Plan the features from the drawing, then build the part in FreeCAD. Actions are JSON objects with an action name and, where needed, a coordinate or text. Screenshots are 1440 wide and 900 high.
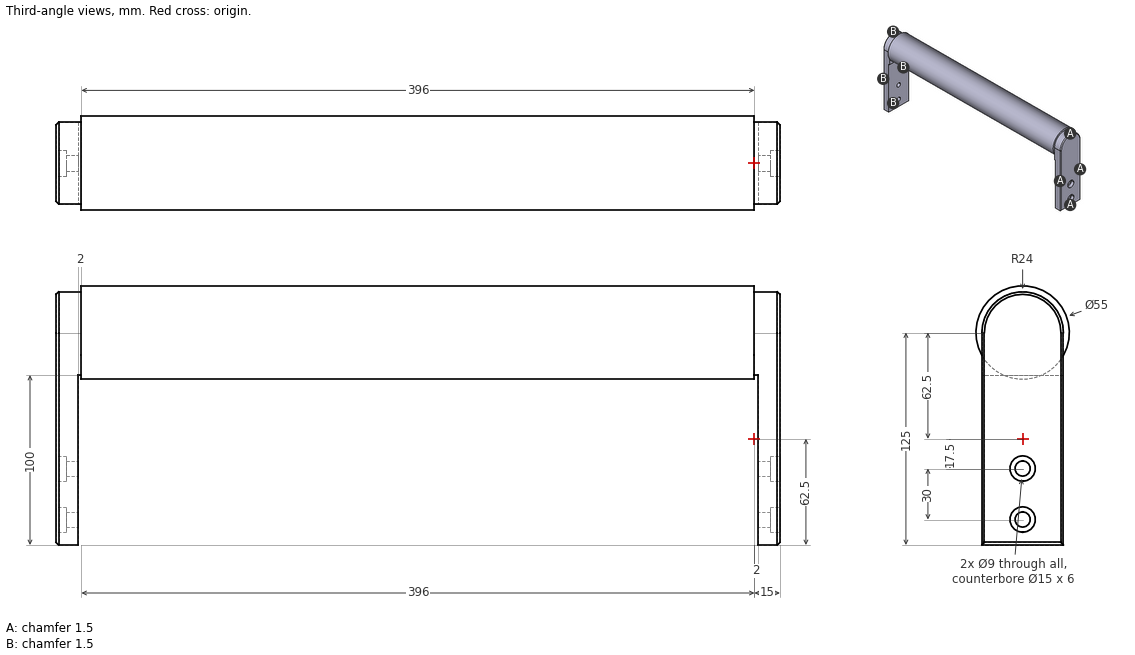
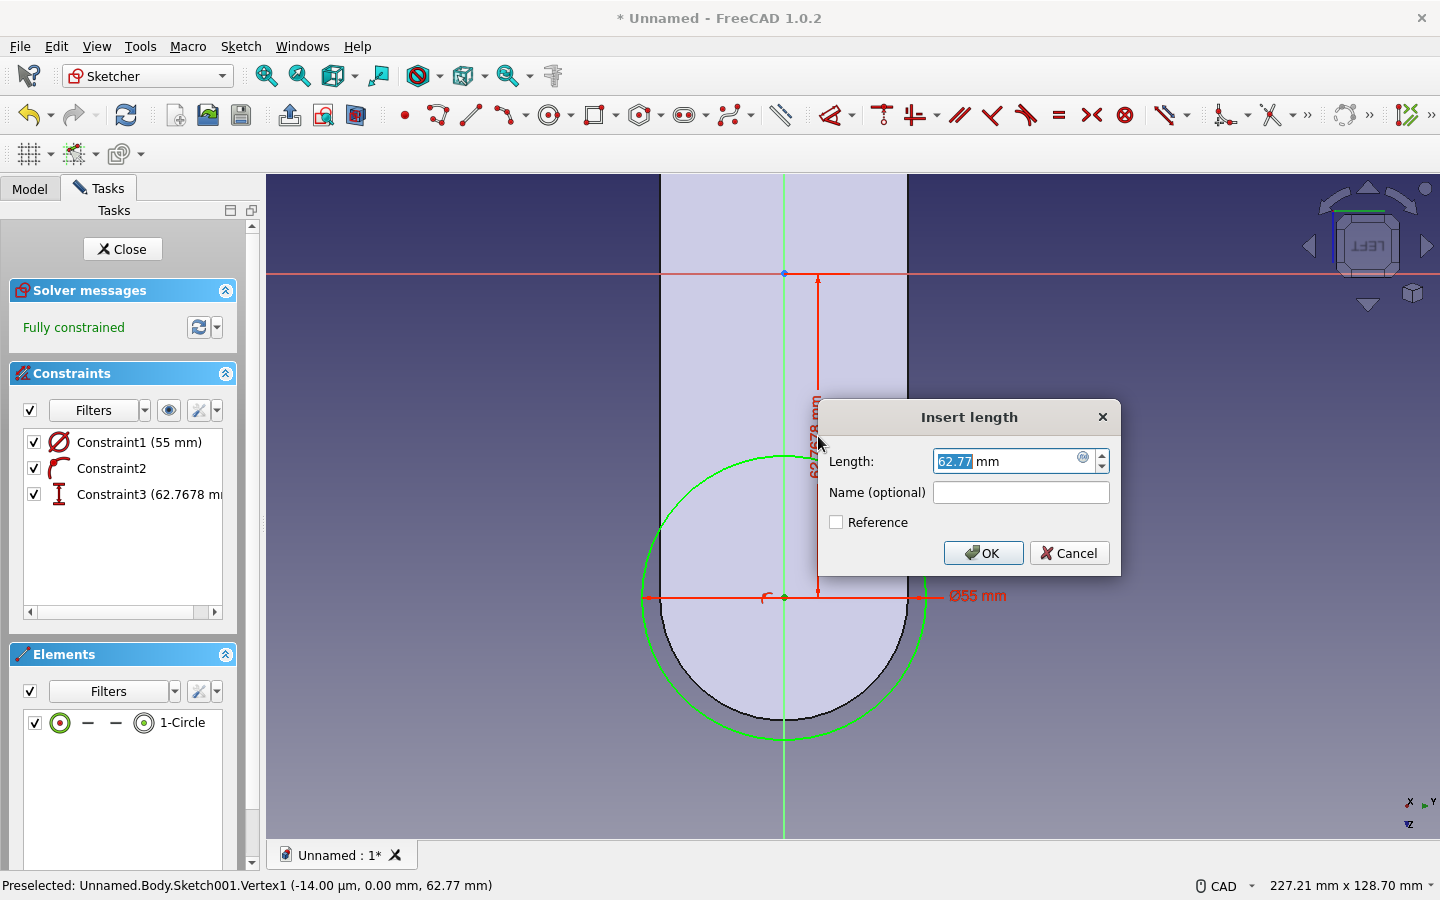
{"action": "type", "text": "62.5"}
{"action": "key", "text": "Return"}
{"action": "key", "text": "Escape"}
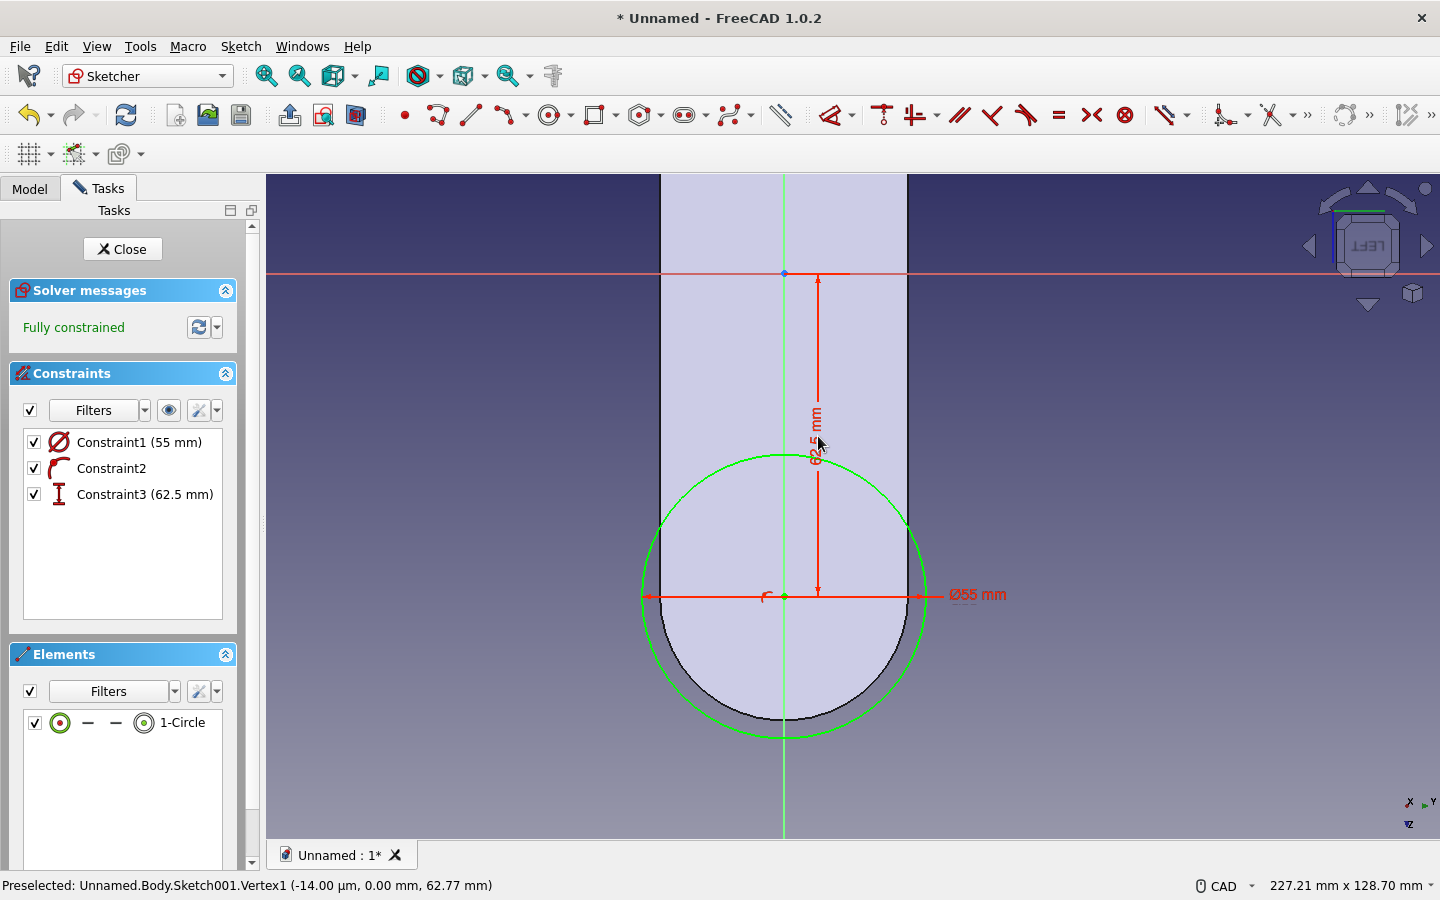
{"action": "left_click", "coordinate": [123, 249]}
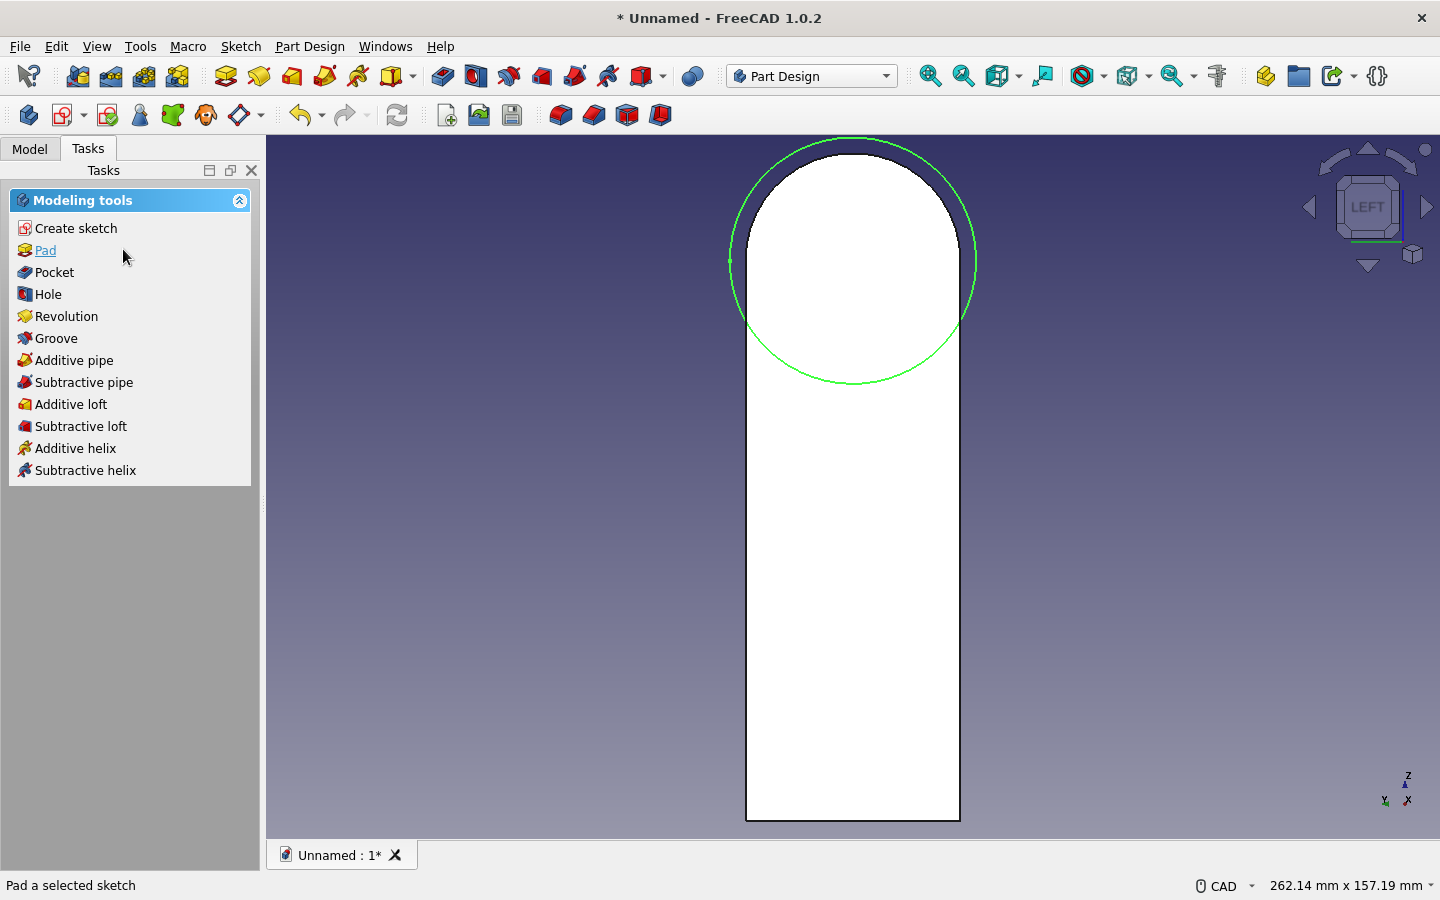
{"action": "left_click", "coordinate": [226, 76]}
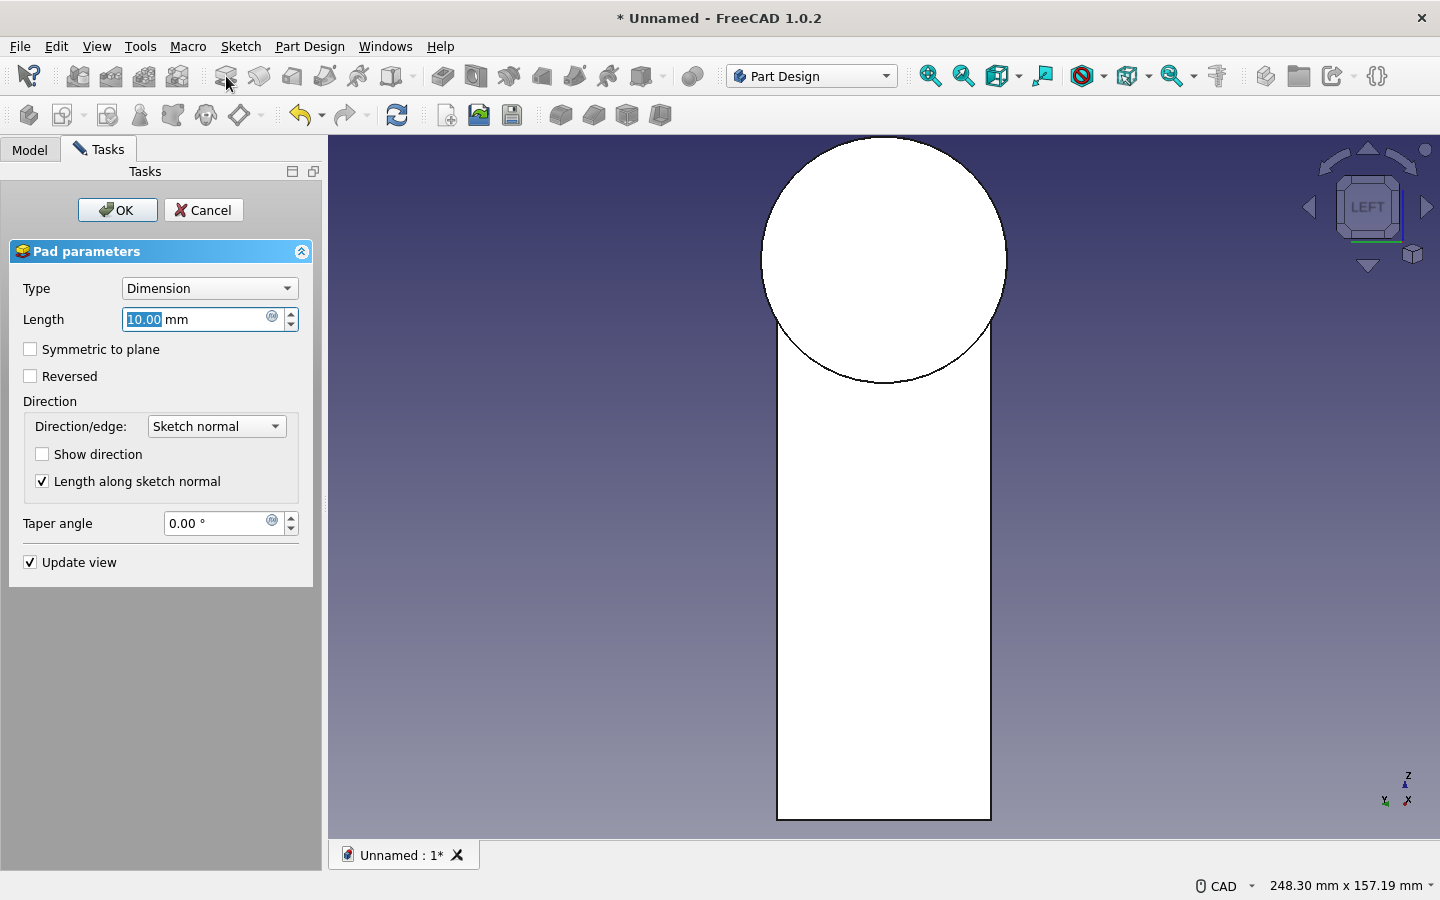
{"action": "type", "text": "396"}
{"action": "key", "text": "Tab"}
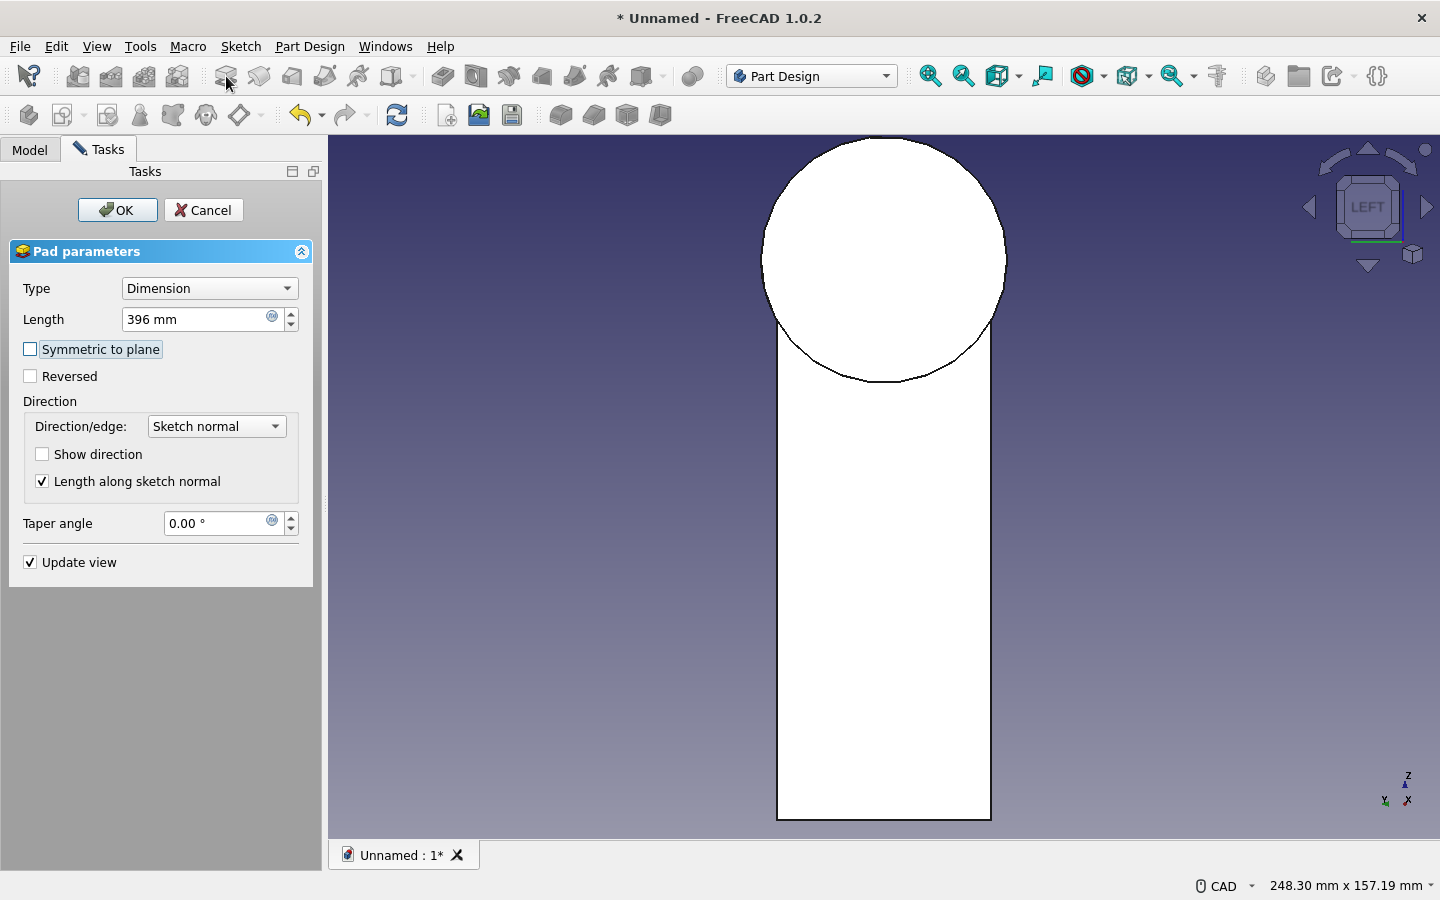
{"action": "left_click", "coordinate": [118, 210]}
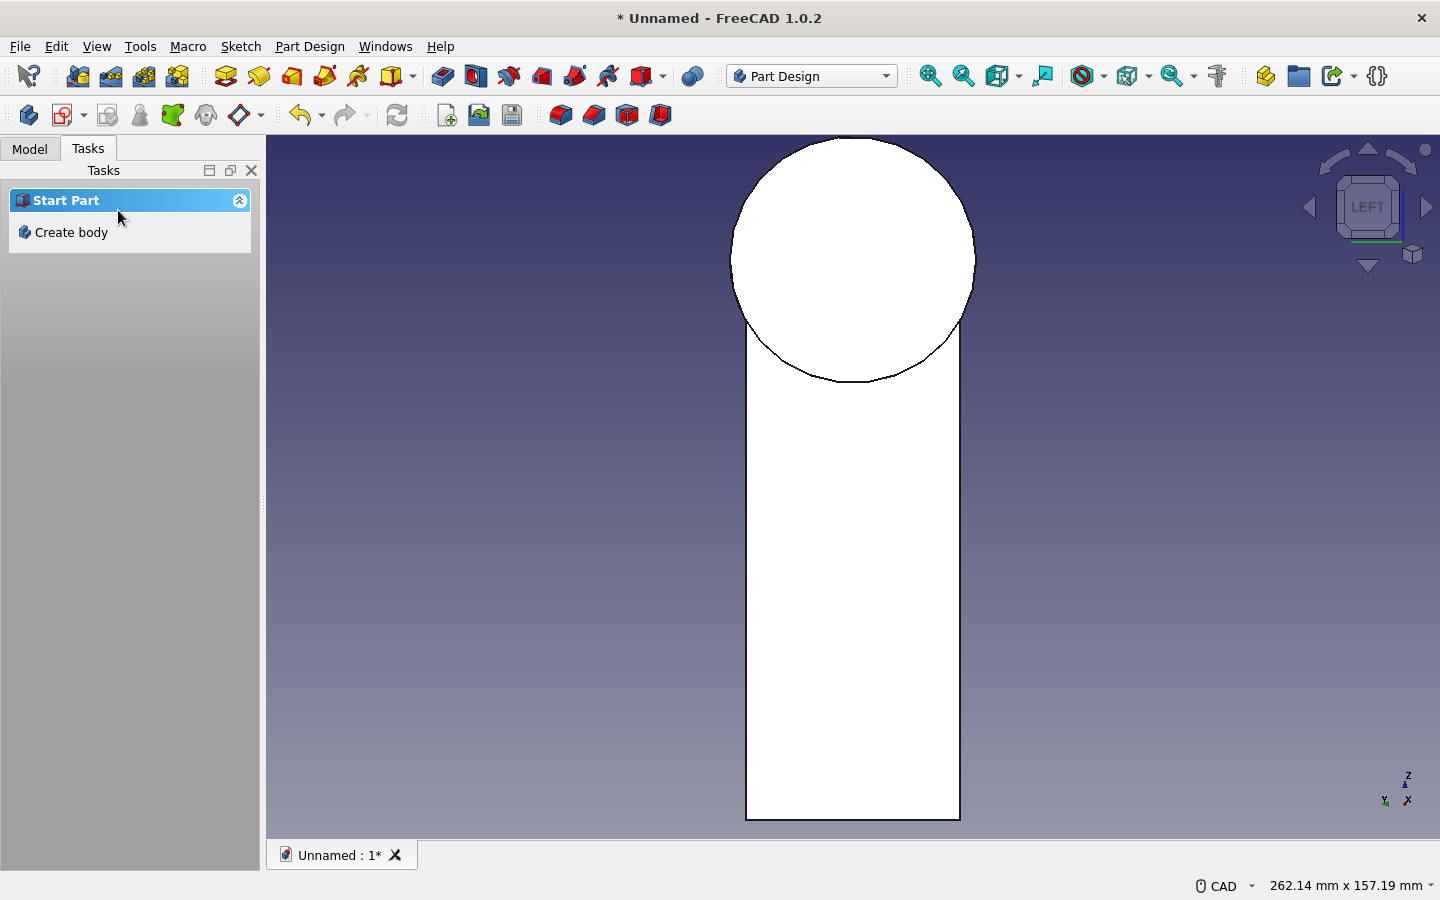
{"action": "key", "text": "0"}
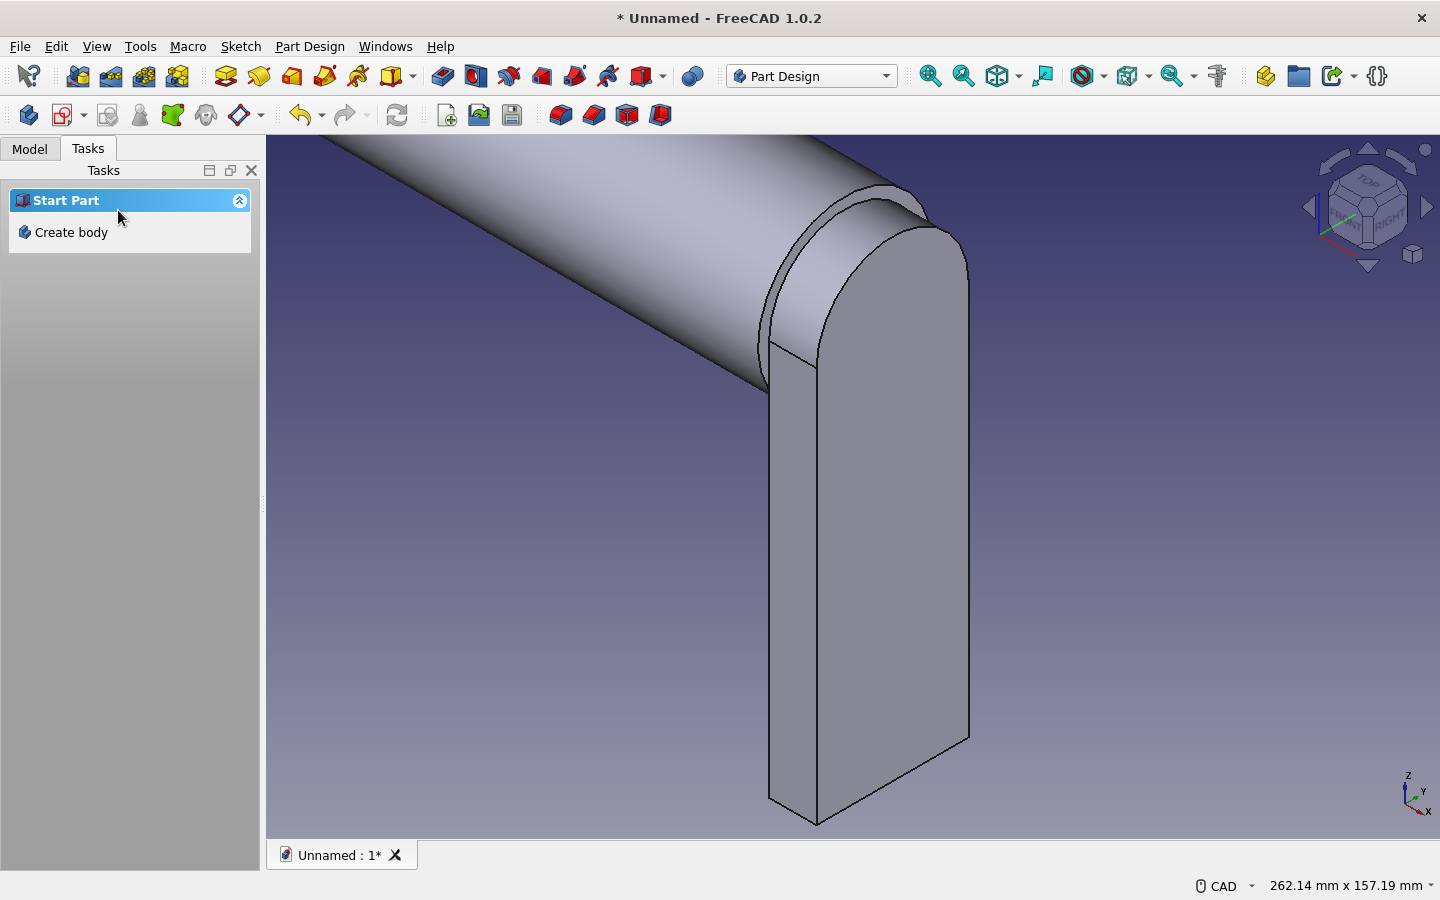
{"action": "left_click", "coordinate": [931, 76]}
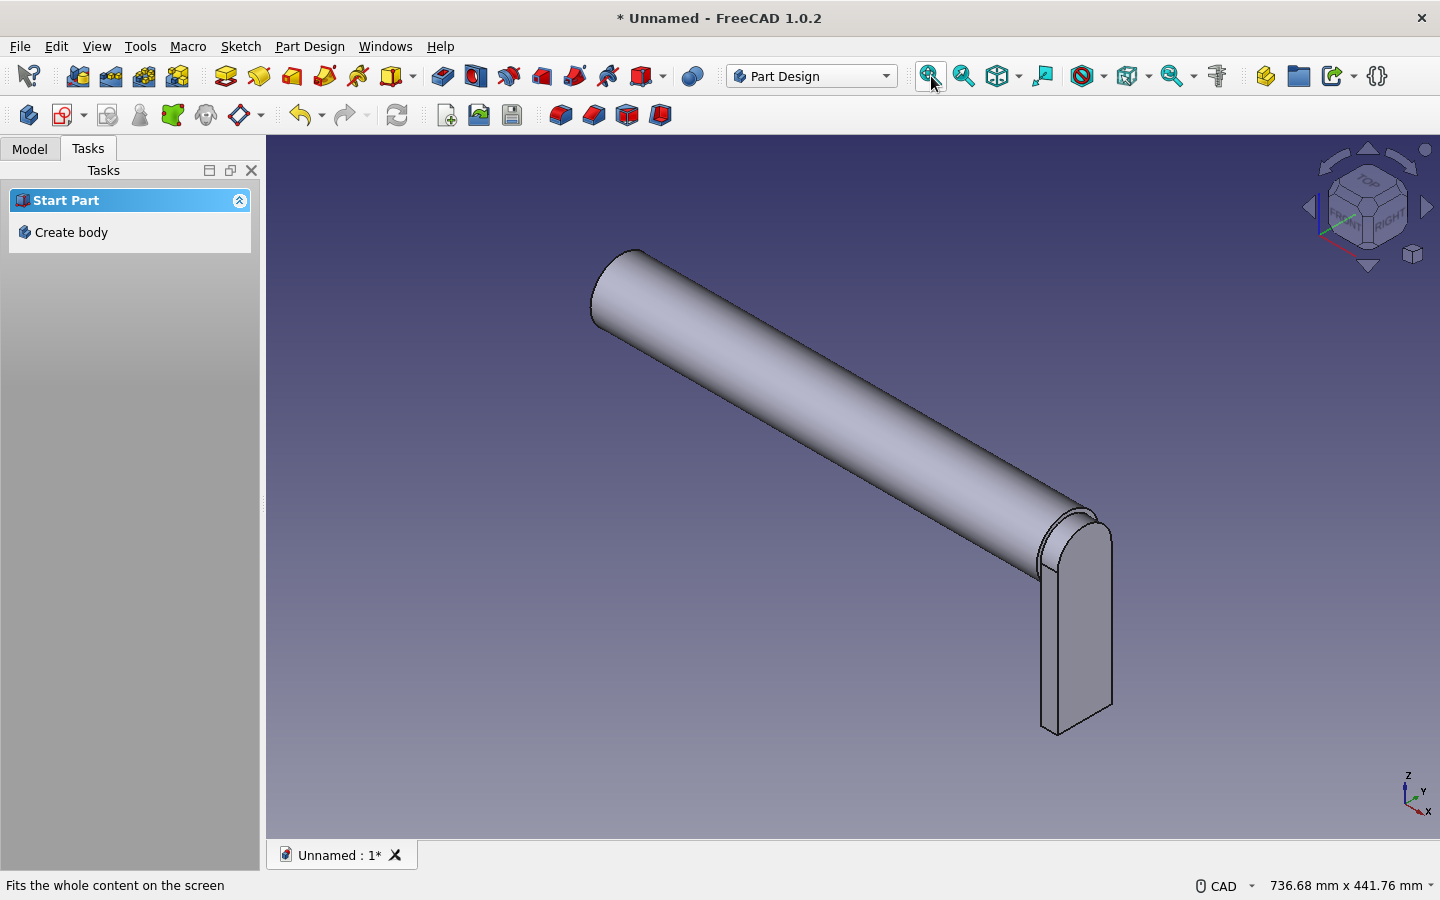
{"action": "left_click", "coordinate": [1085, 677]}